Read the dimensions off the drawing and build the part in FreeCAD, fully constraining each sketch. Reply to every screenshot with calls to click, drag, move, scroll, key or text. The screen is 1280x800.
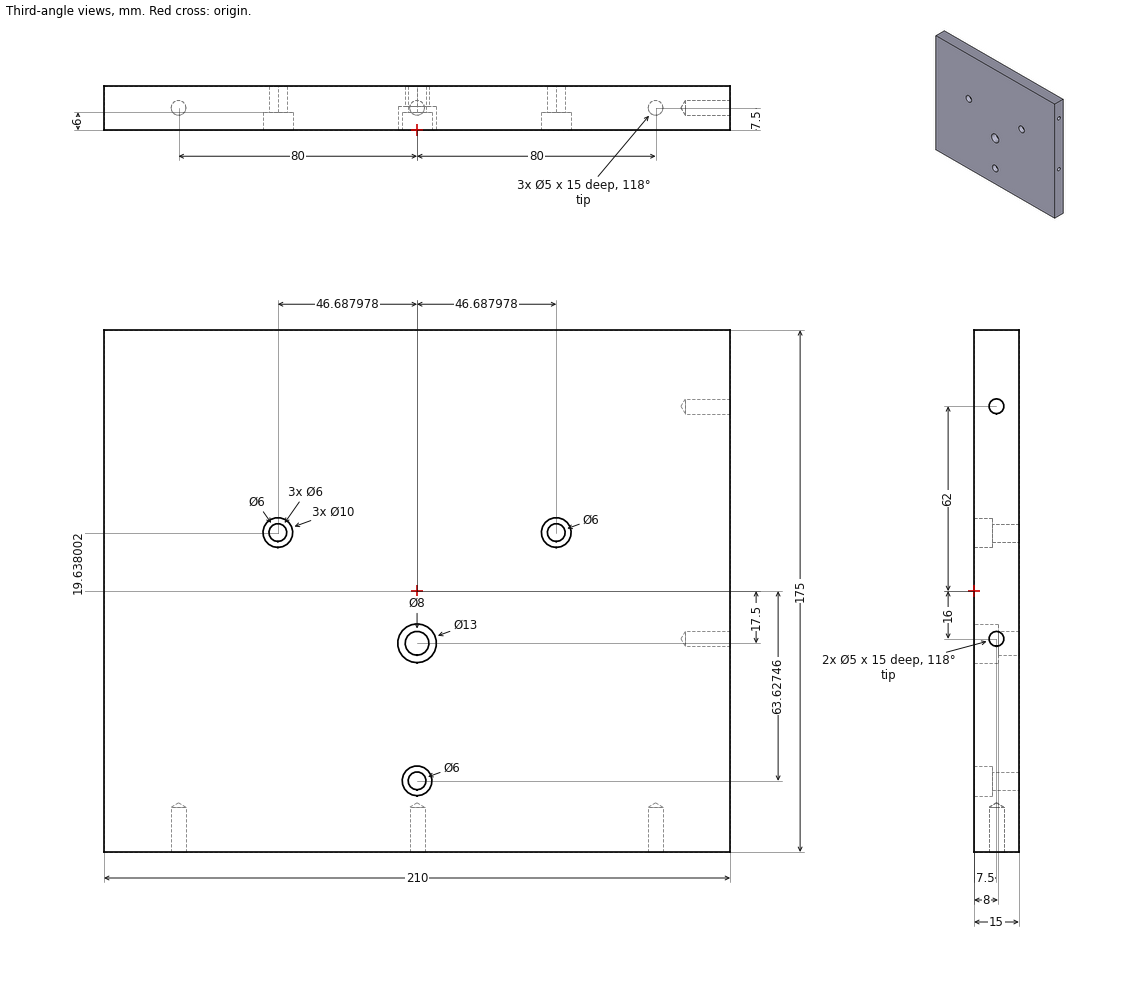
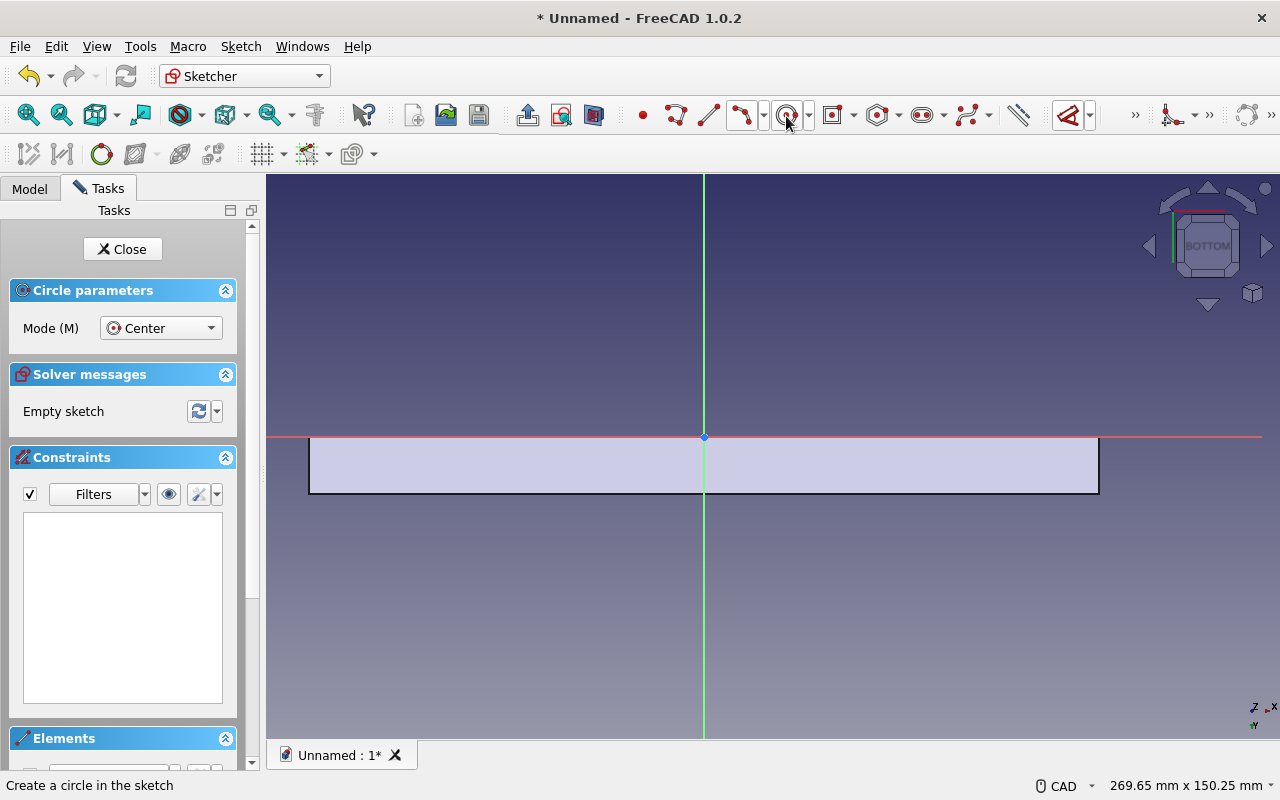
scroll(1005, 466, up, 5)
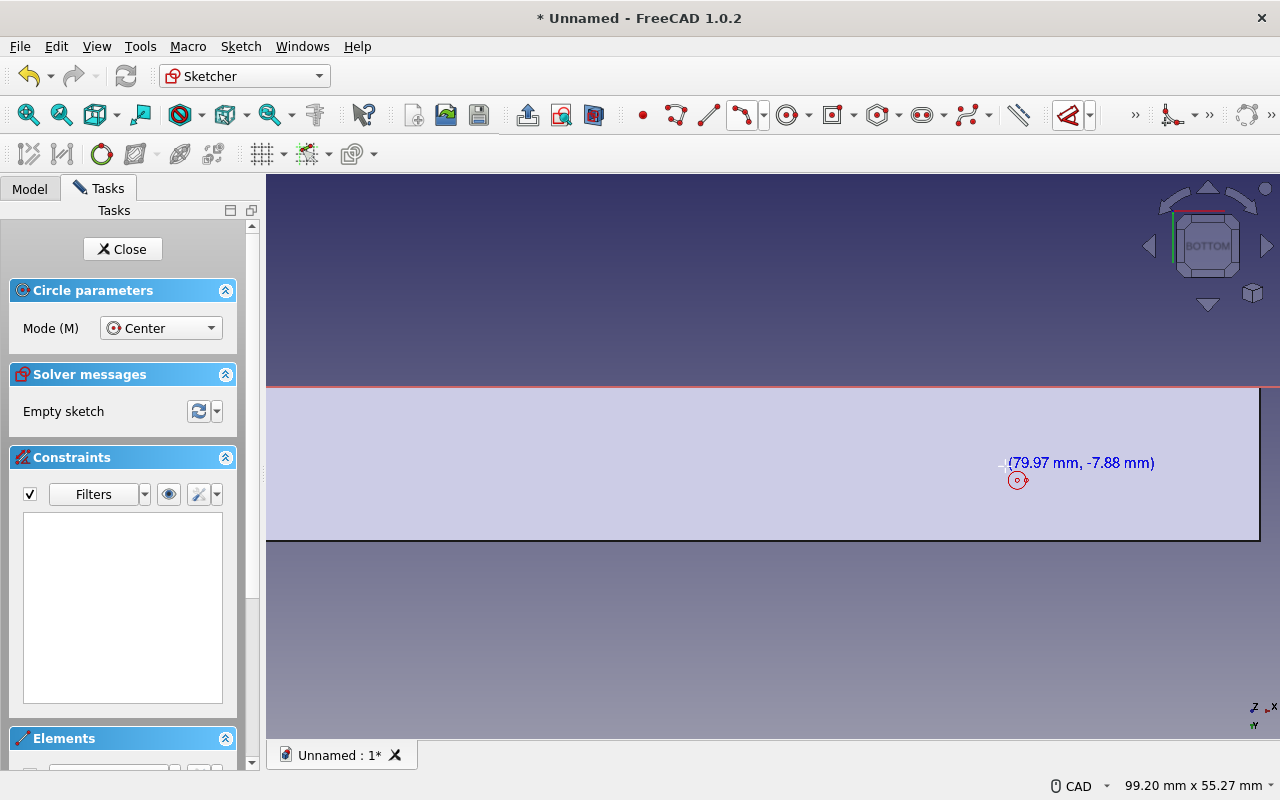
click(1004, 464)
click(1022, 446)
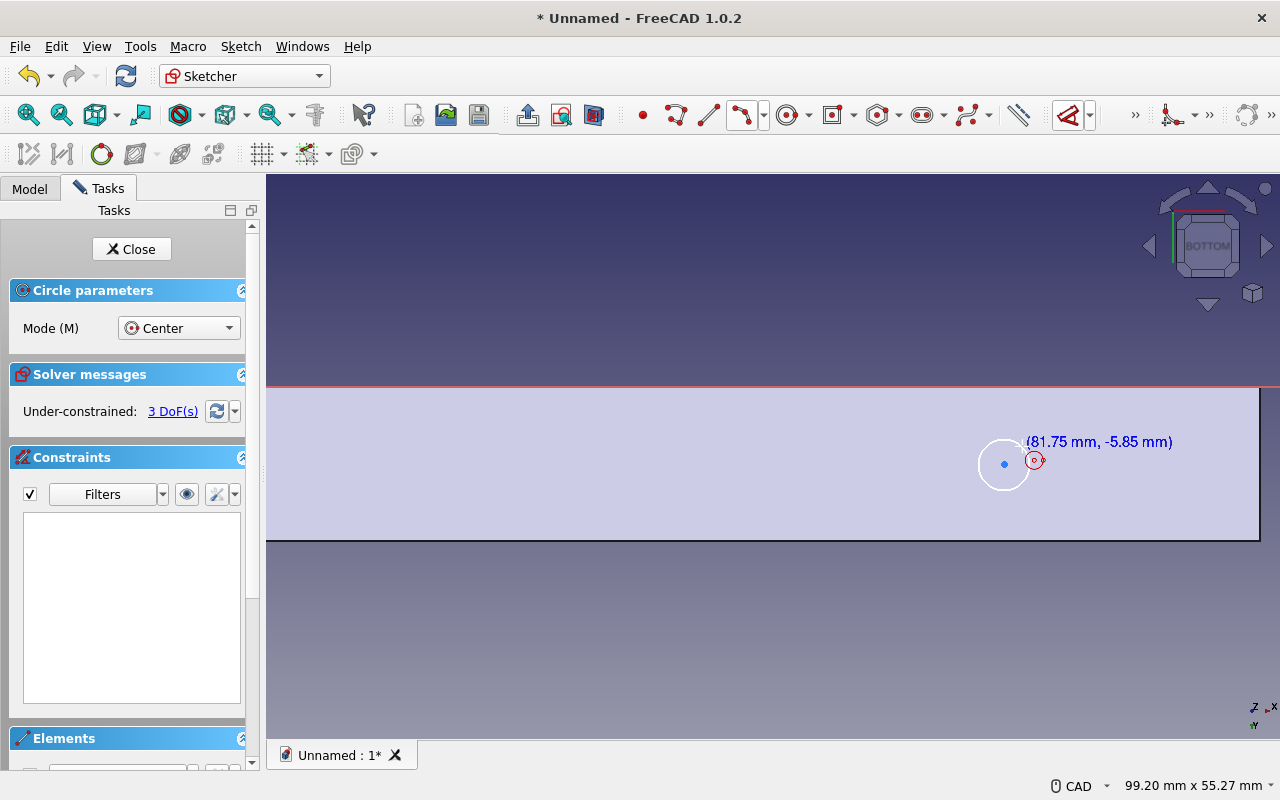
scroll(1006, 467, down, 5)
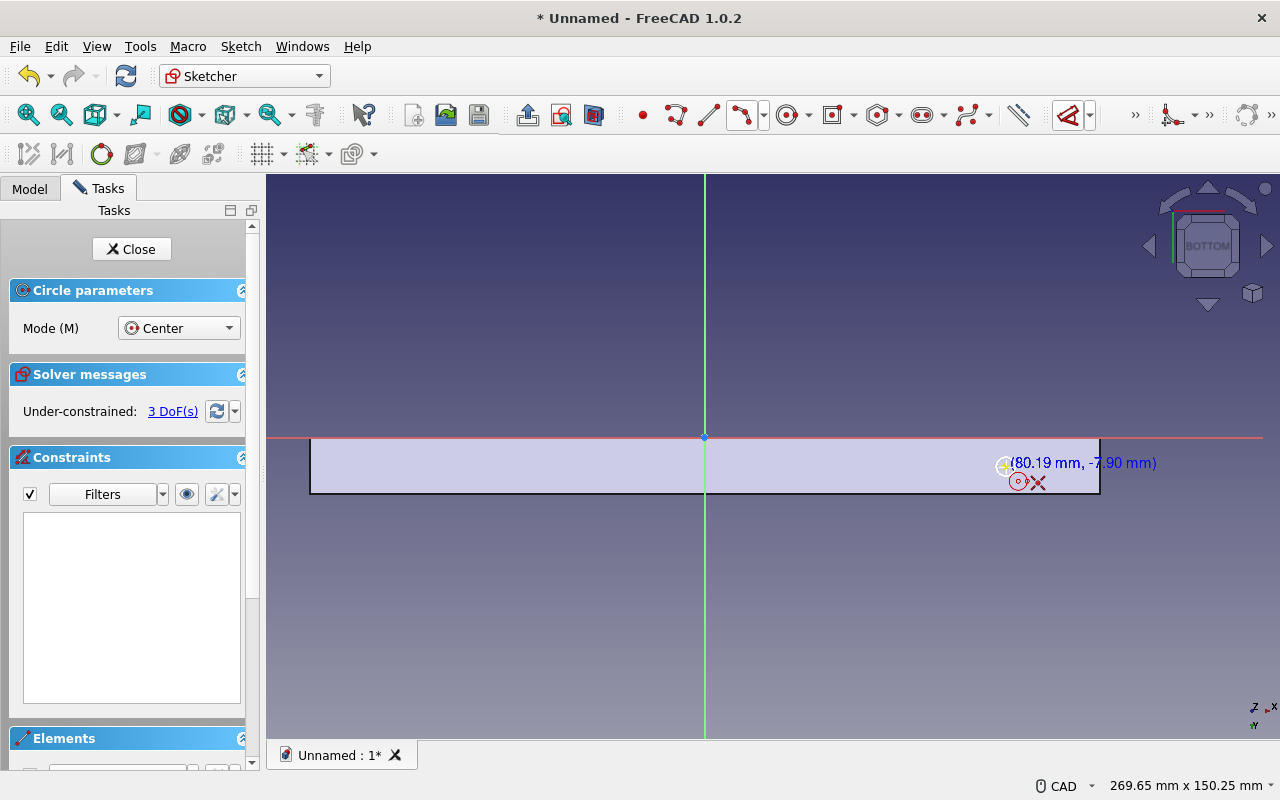
scroll(705, 466, up, 5)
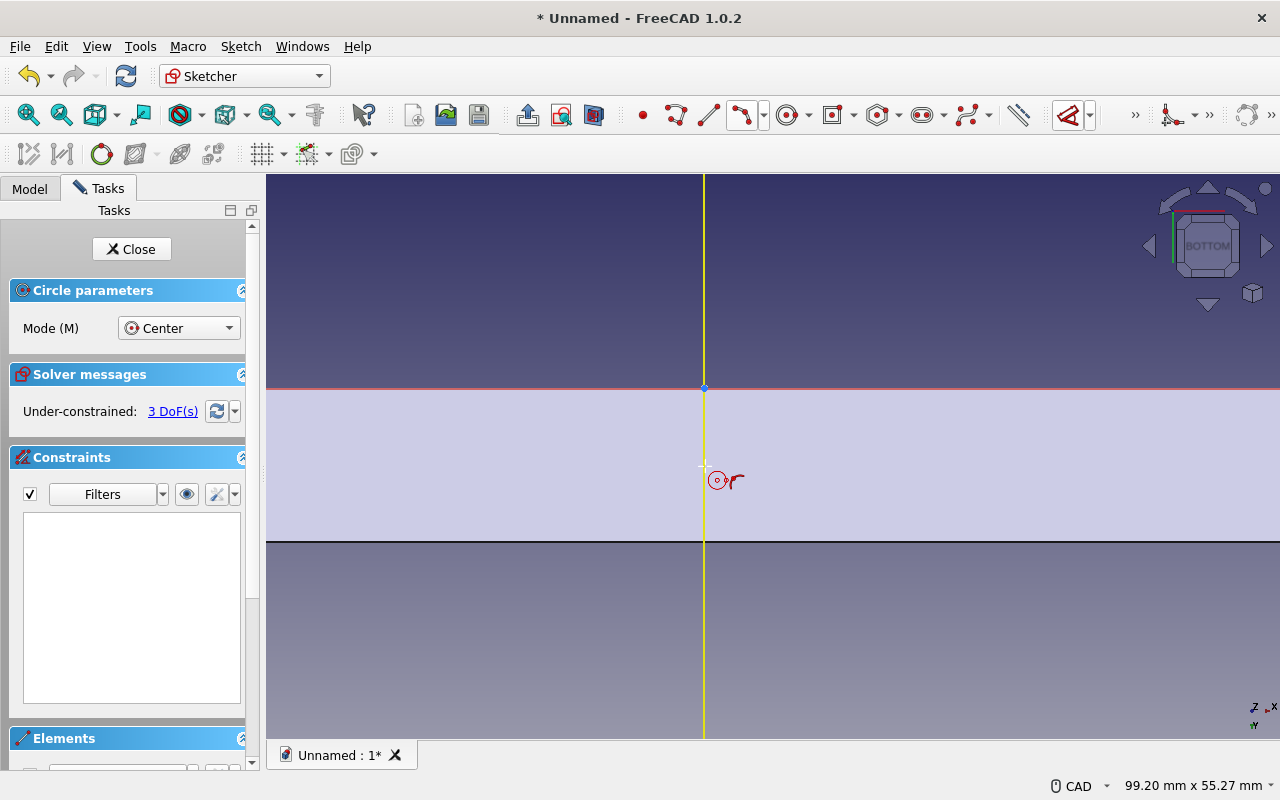
click(704, 466)
click(722, 448)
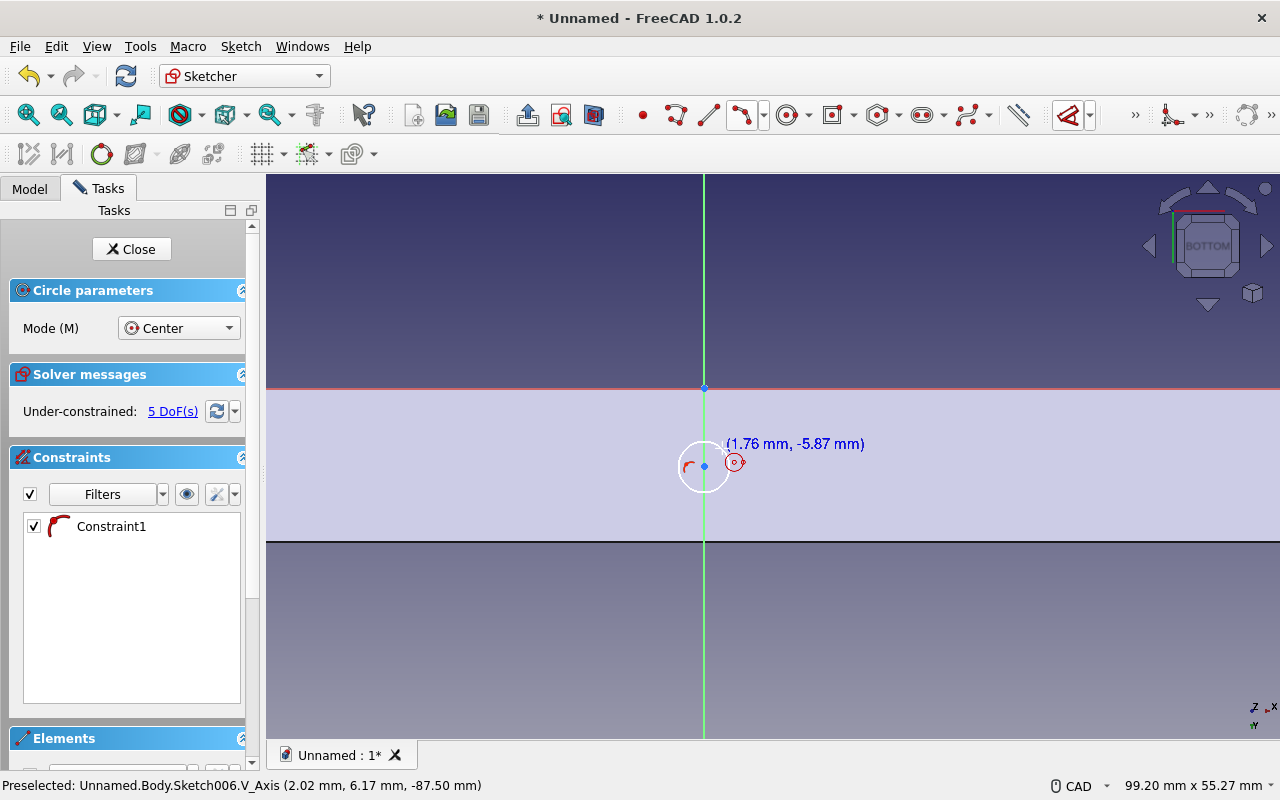
scroll(705, 466, down, 5)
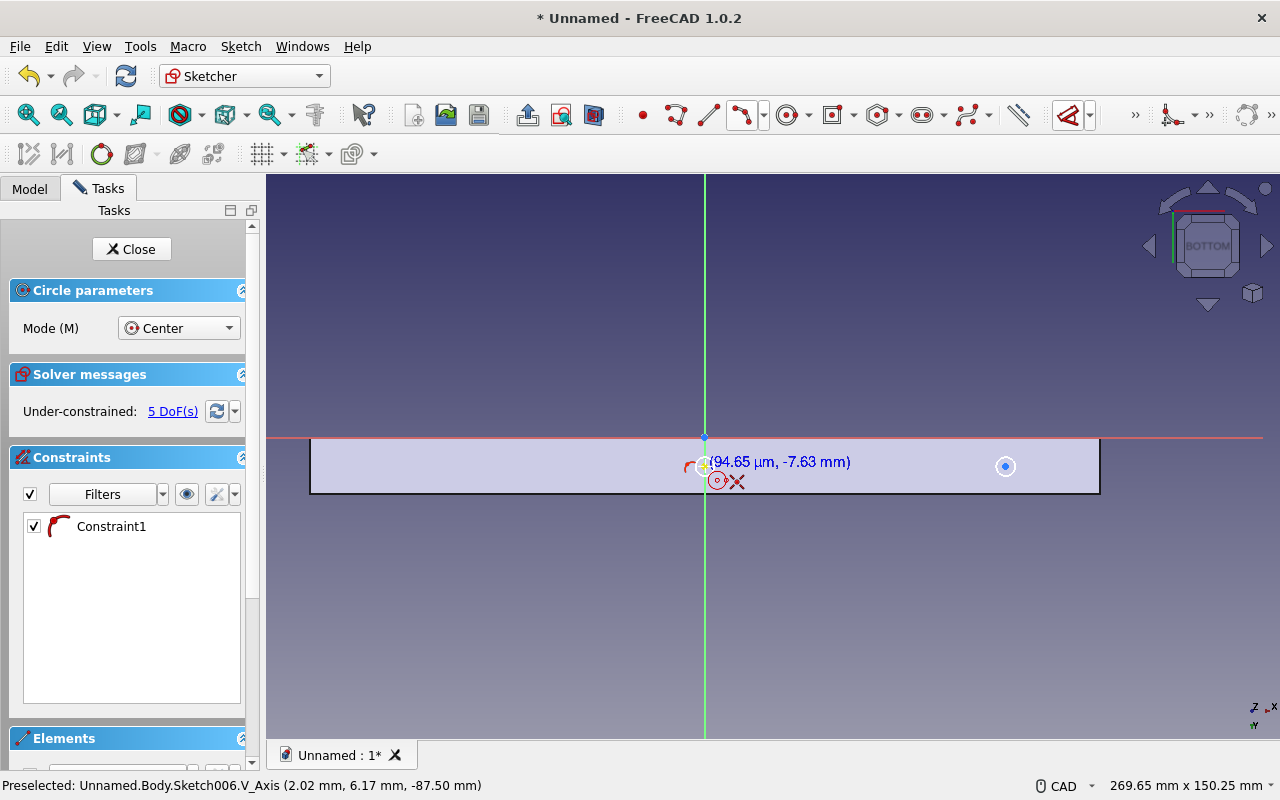
scroll(404, 466, up, 5)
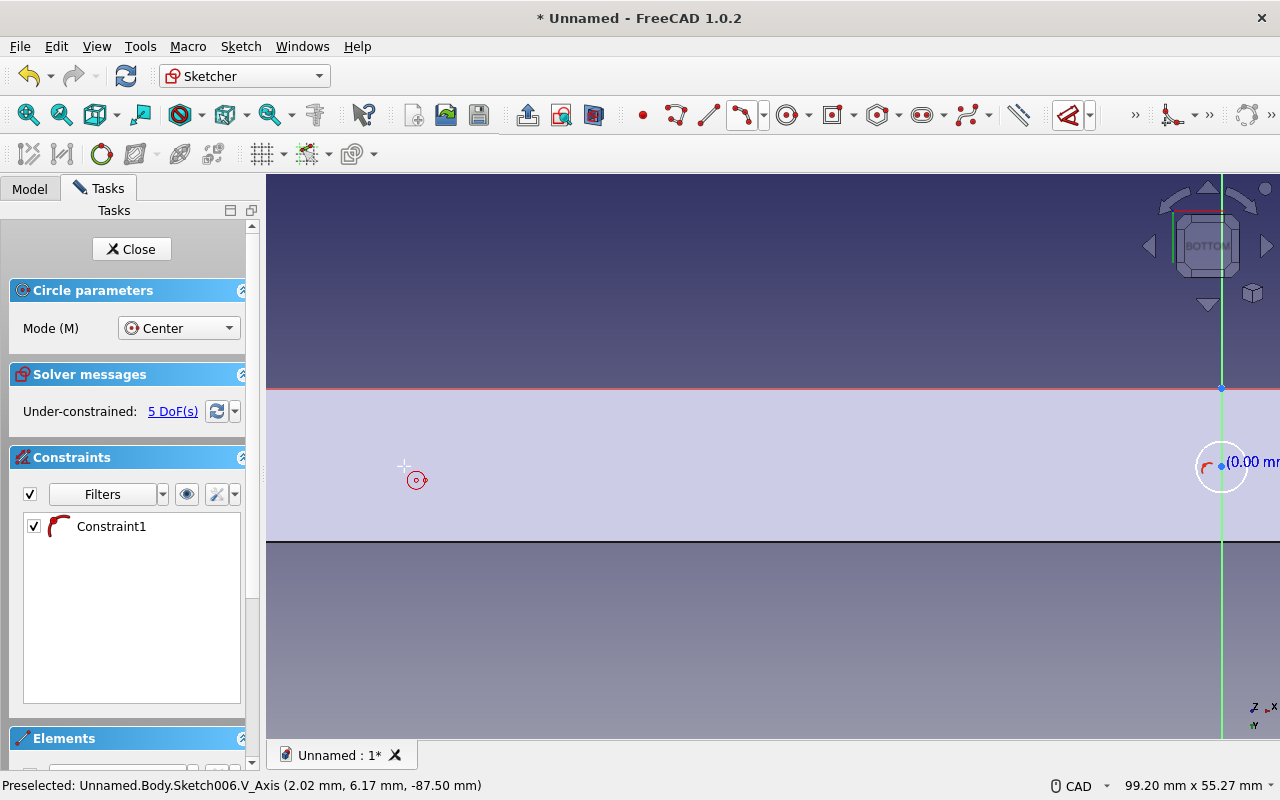
click(404, 466)
click(422, 448)
key(Escape)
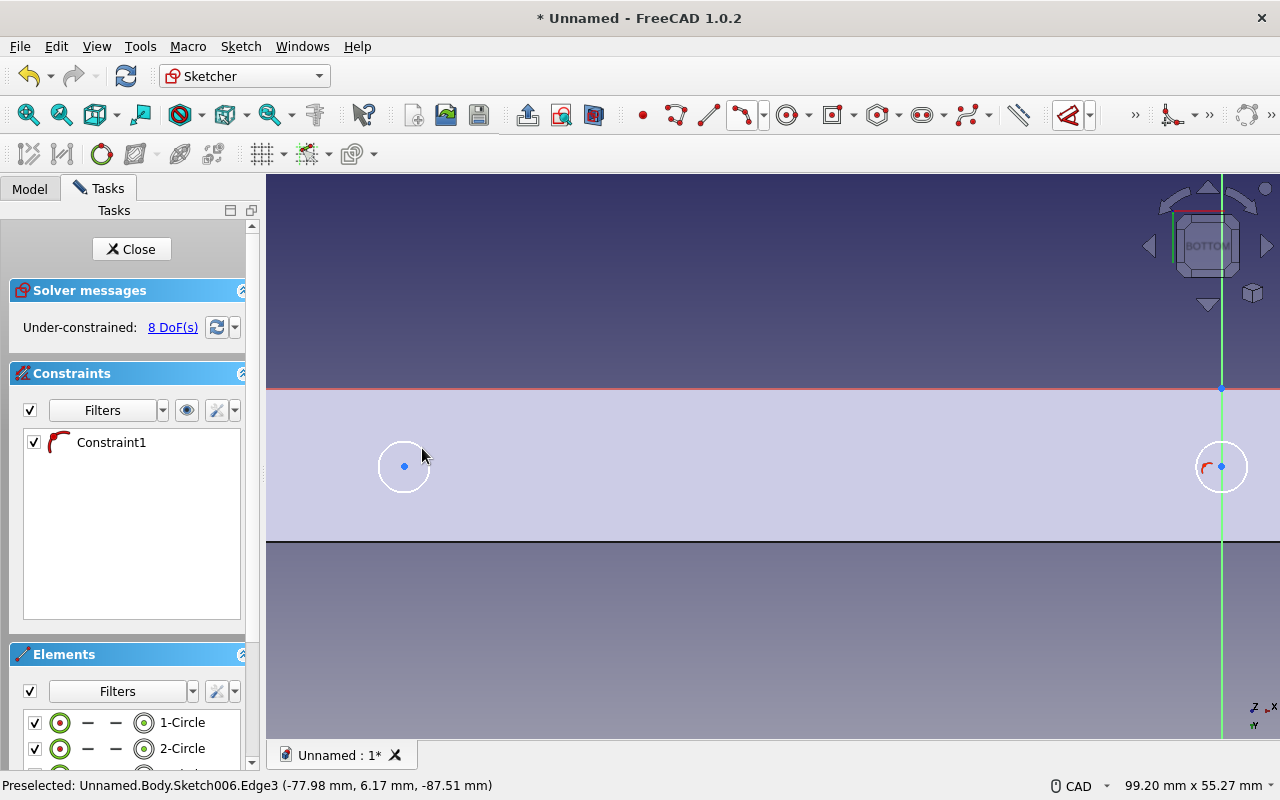
scroll(403, 466, down, 5)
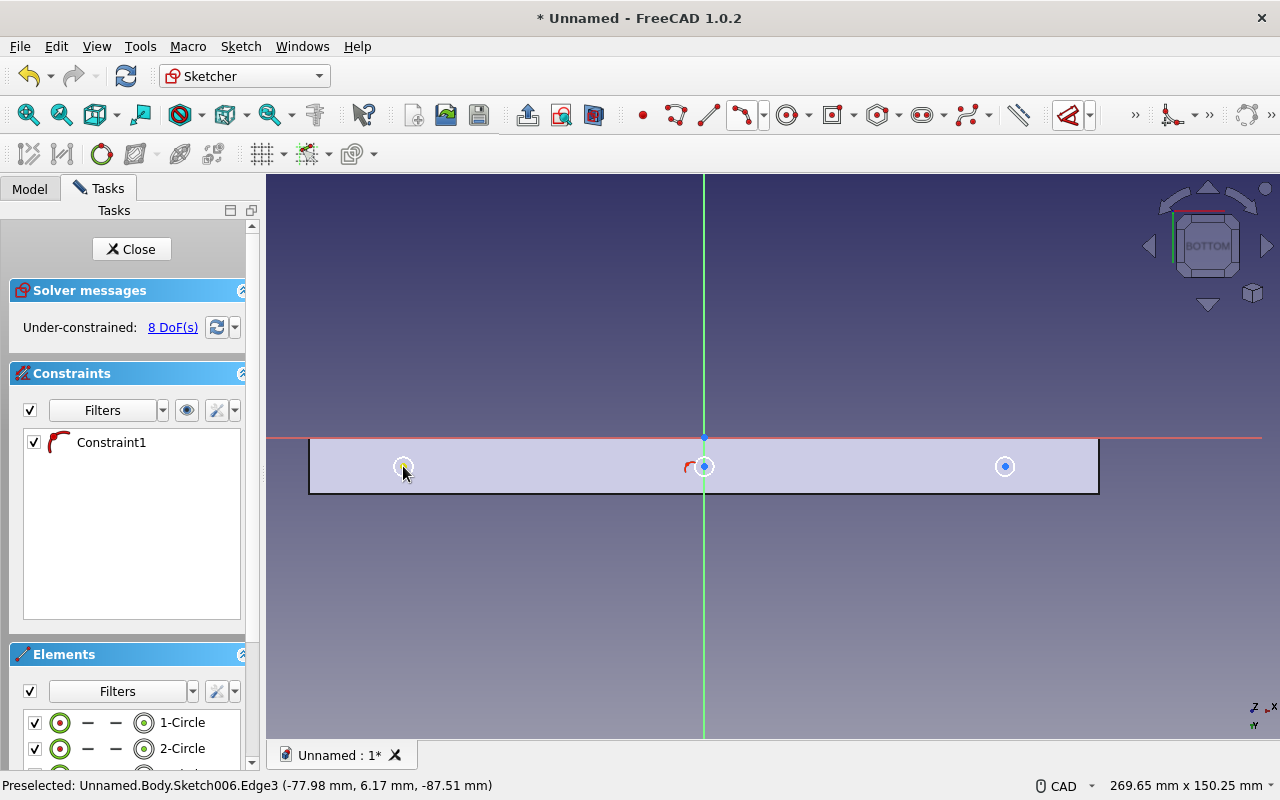
scroll(1012, 460, up, 2)